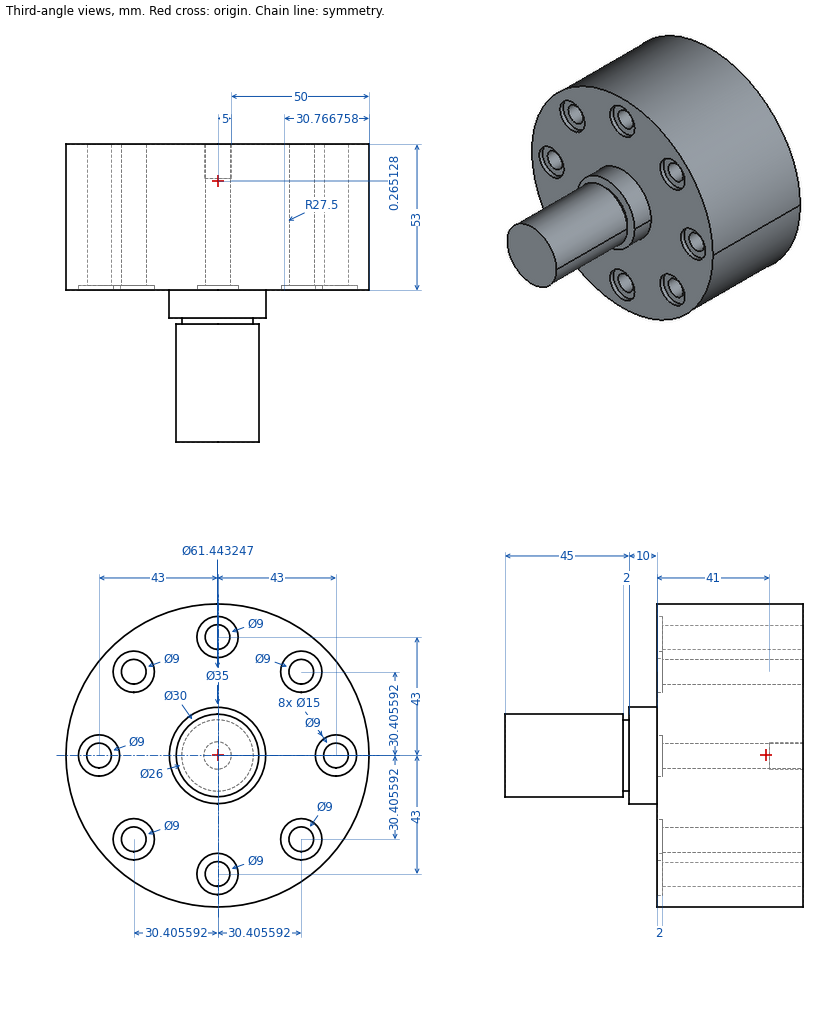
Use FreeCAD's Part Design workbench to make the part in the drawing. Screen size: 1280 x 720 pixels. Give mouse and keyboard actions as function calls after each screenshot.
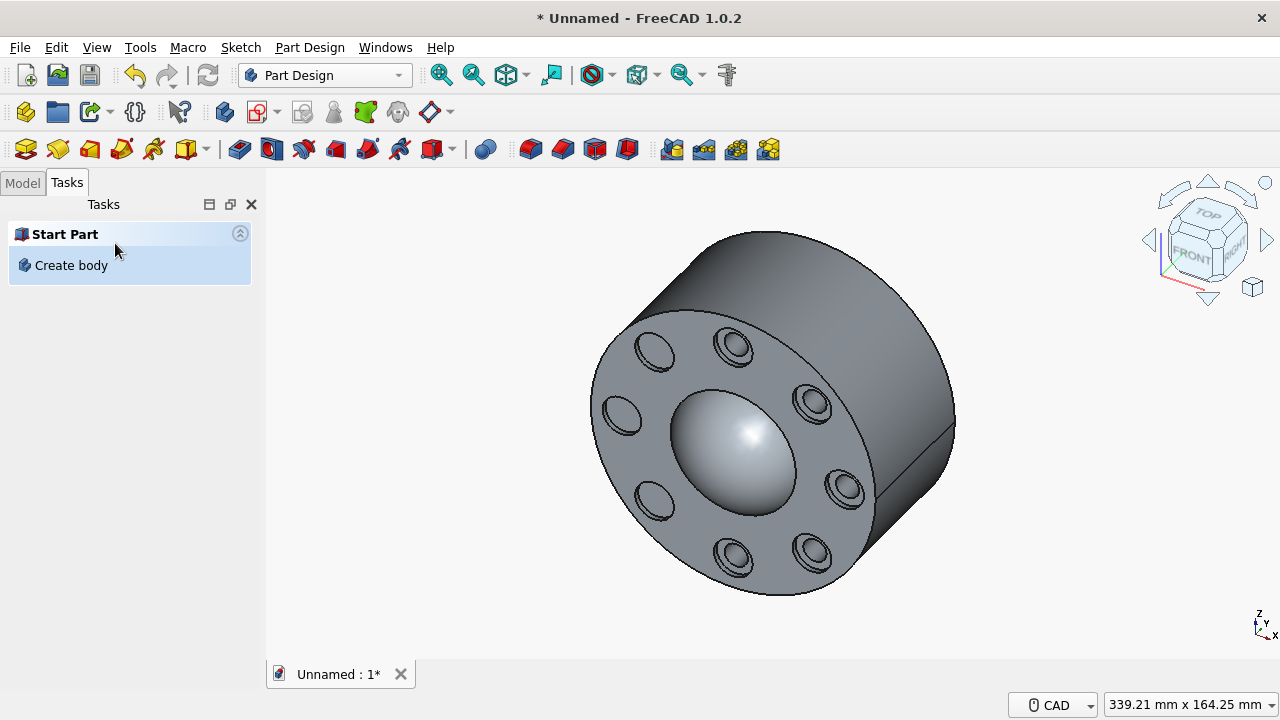
click(658, 348)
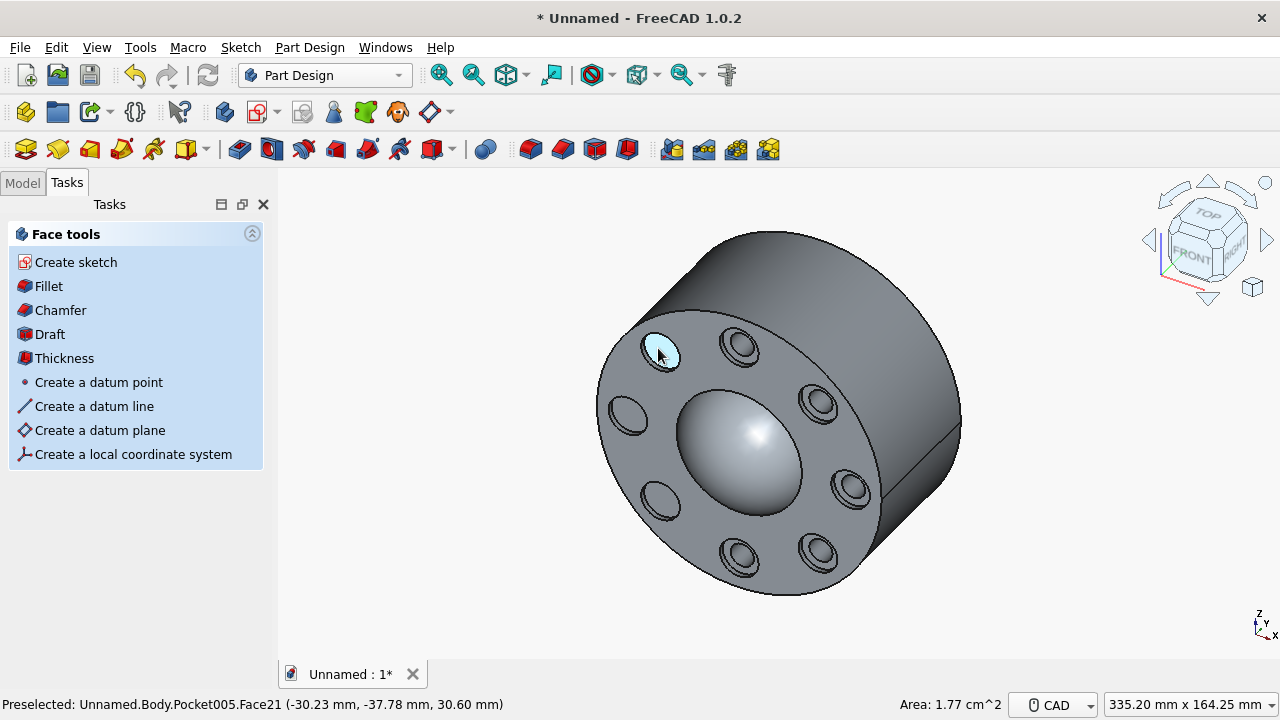
click(258, 112)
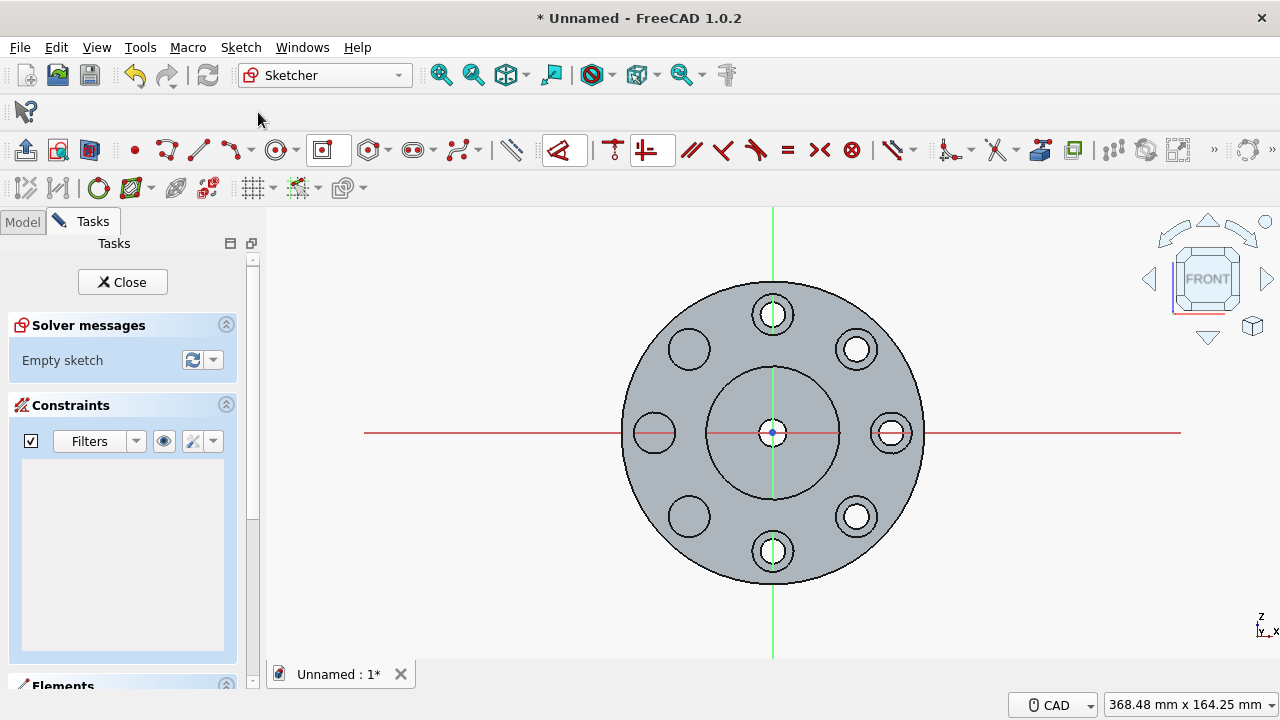
scroll(688, 525, up, 12)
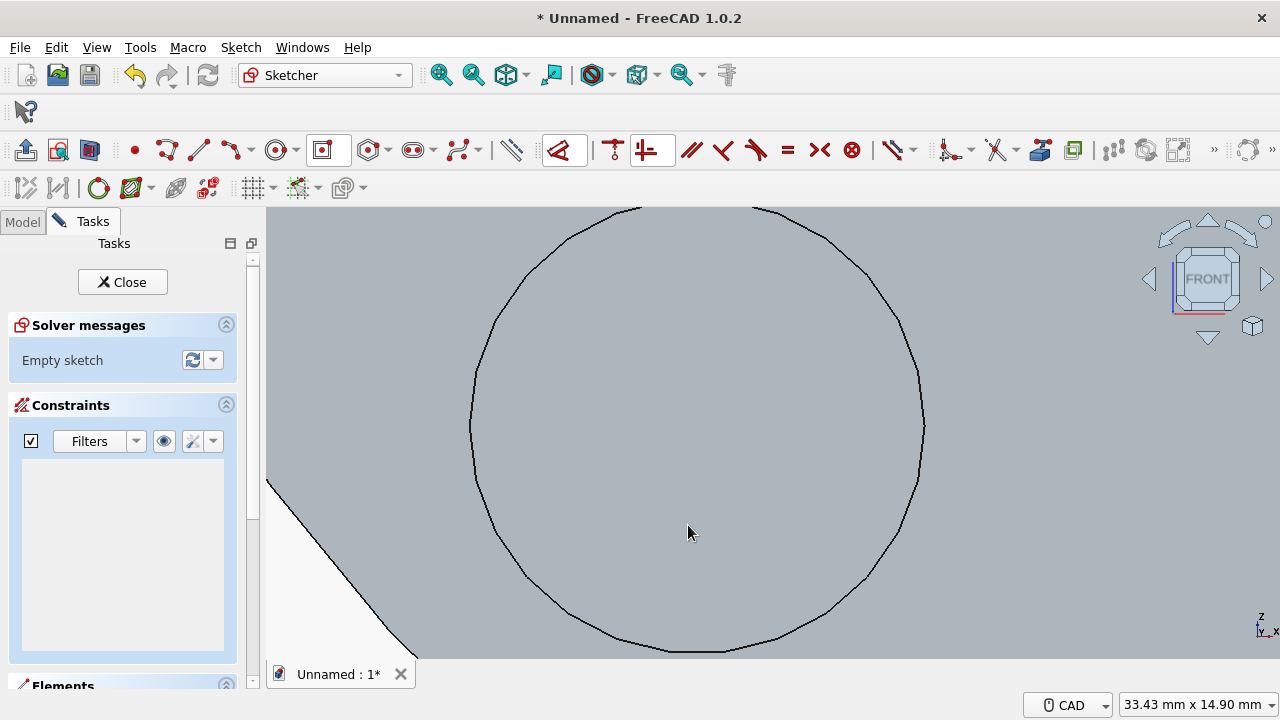
click(276, 150)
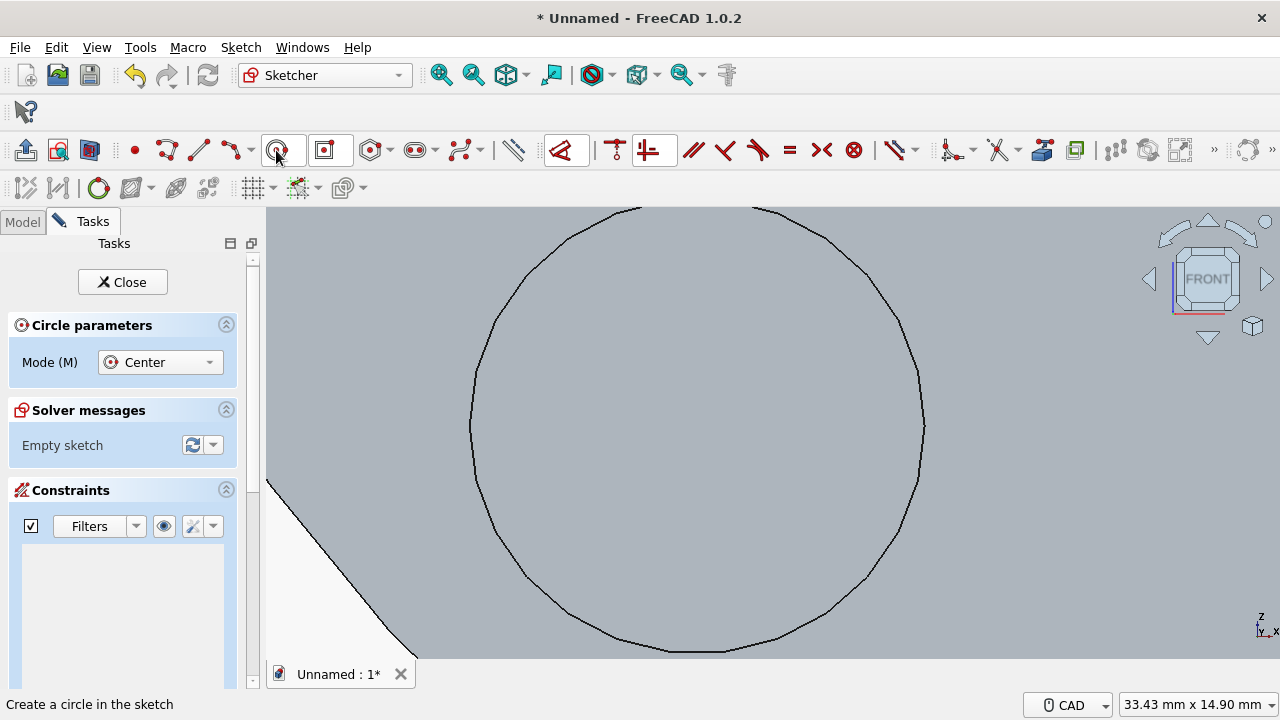
click(697, 426)
move(794, 330)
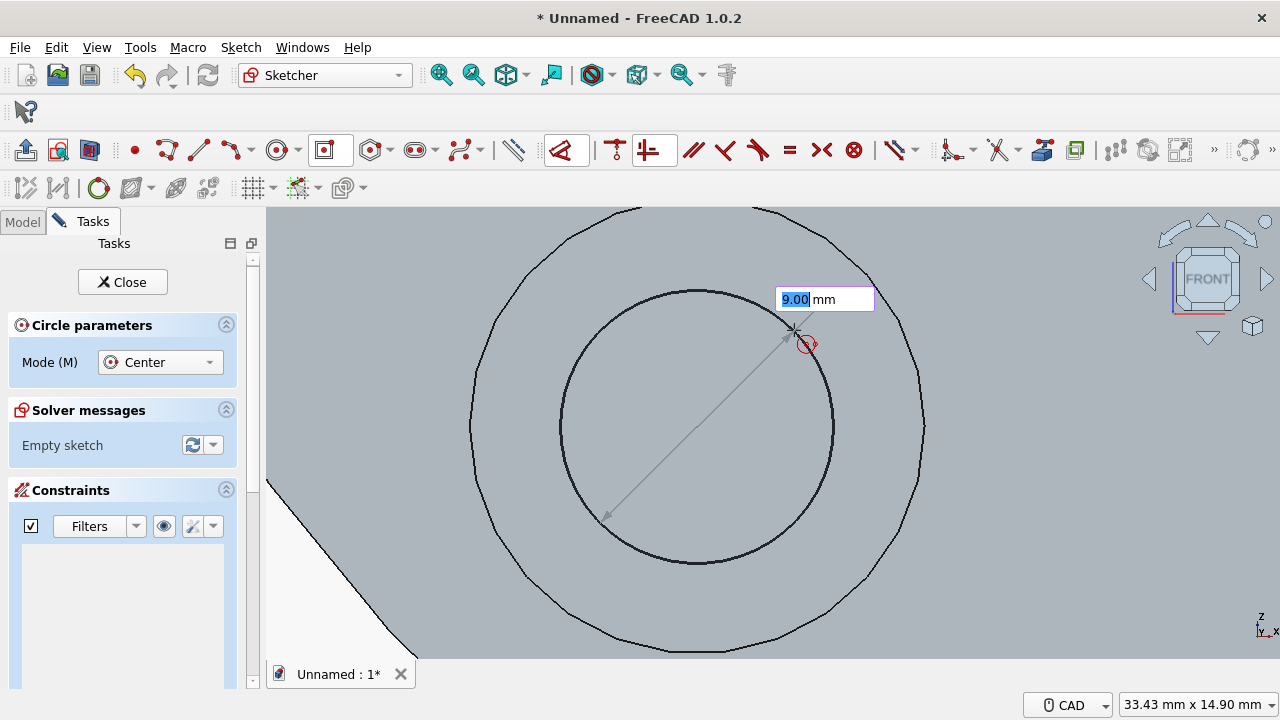
text(9)
key(Return)
key(Escape)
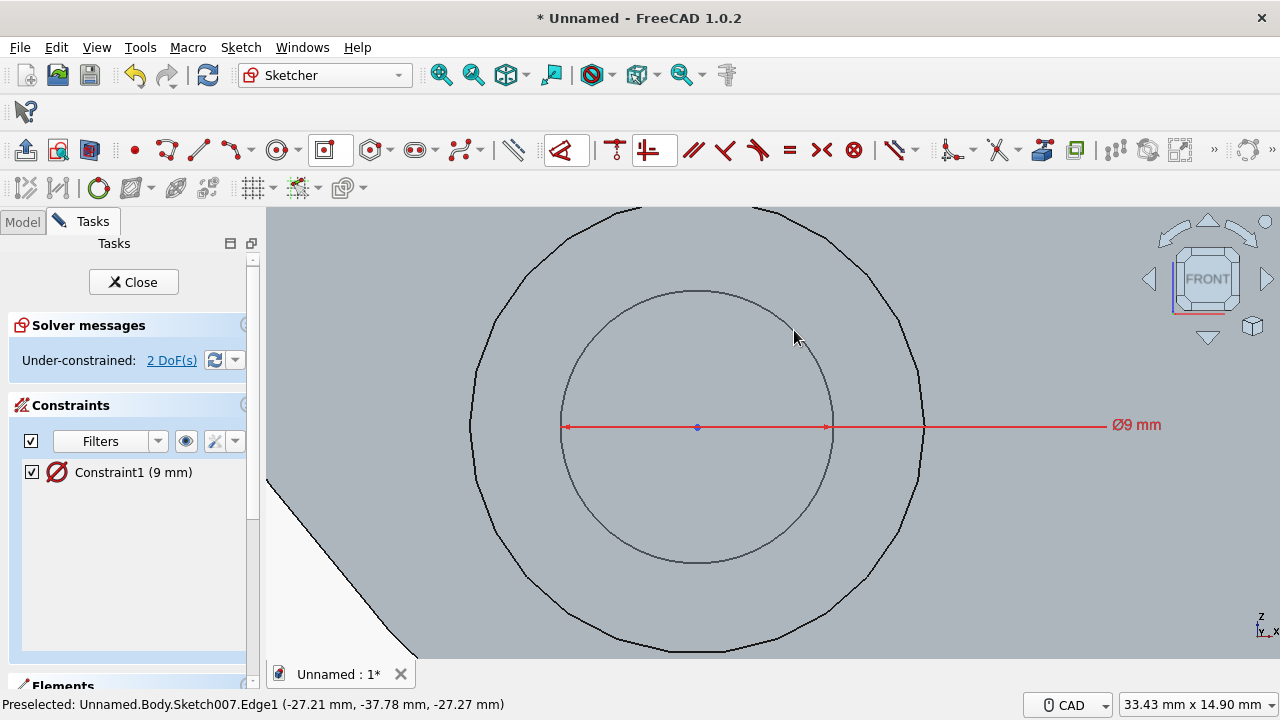
click(697, 427)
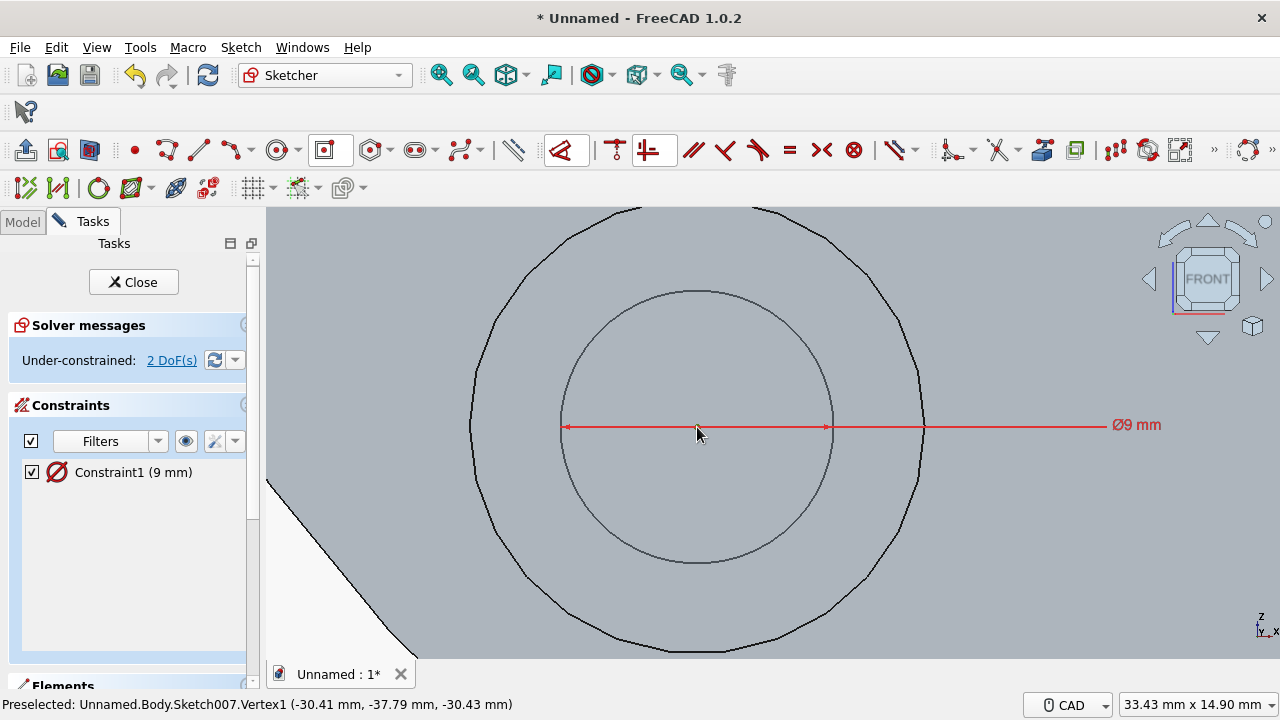
key(l)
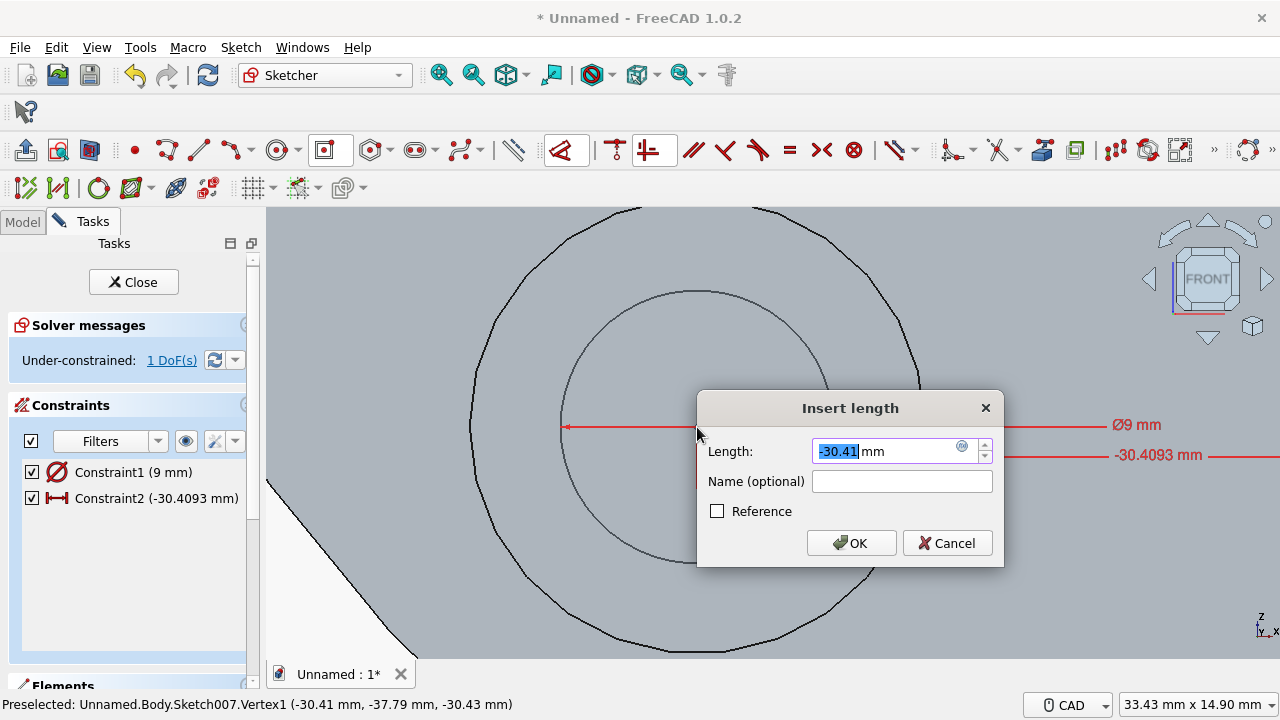
text(-30.405592)
key(Return)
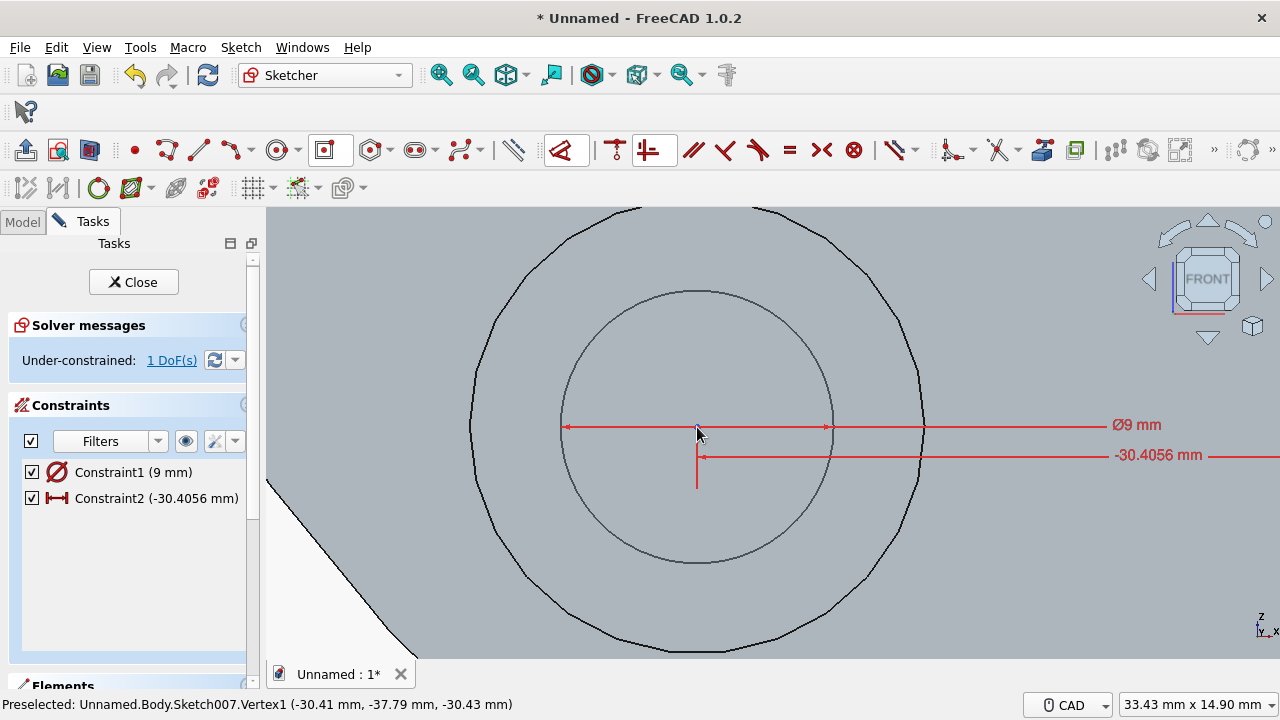
click(697, 427)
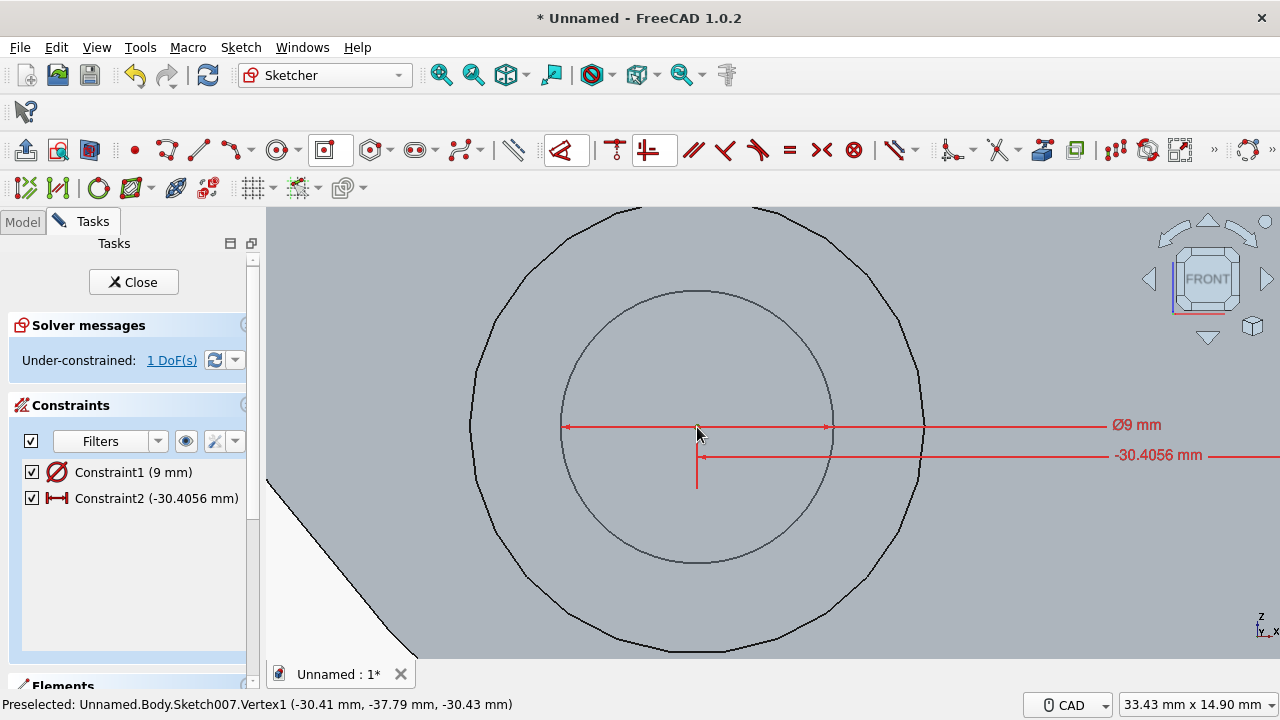
key(i)